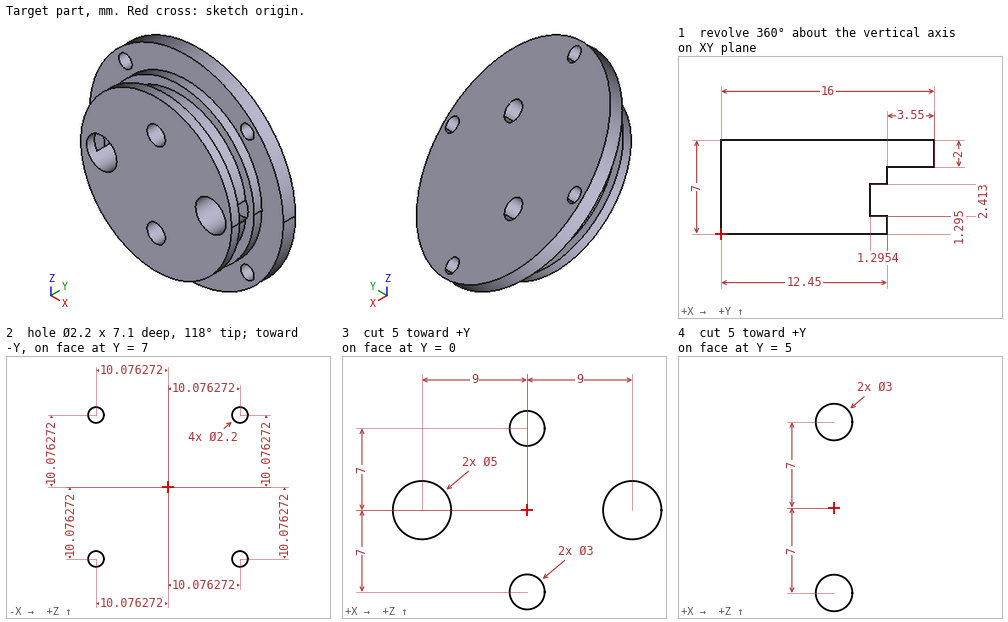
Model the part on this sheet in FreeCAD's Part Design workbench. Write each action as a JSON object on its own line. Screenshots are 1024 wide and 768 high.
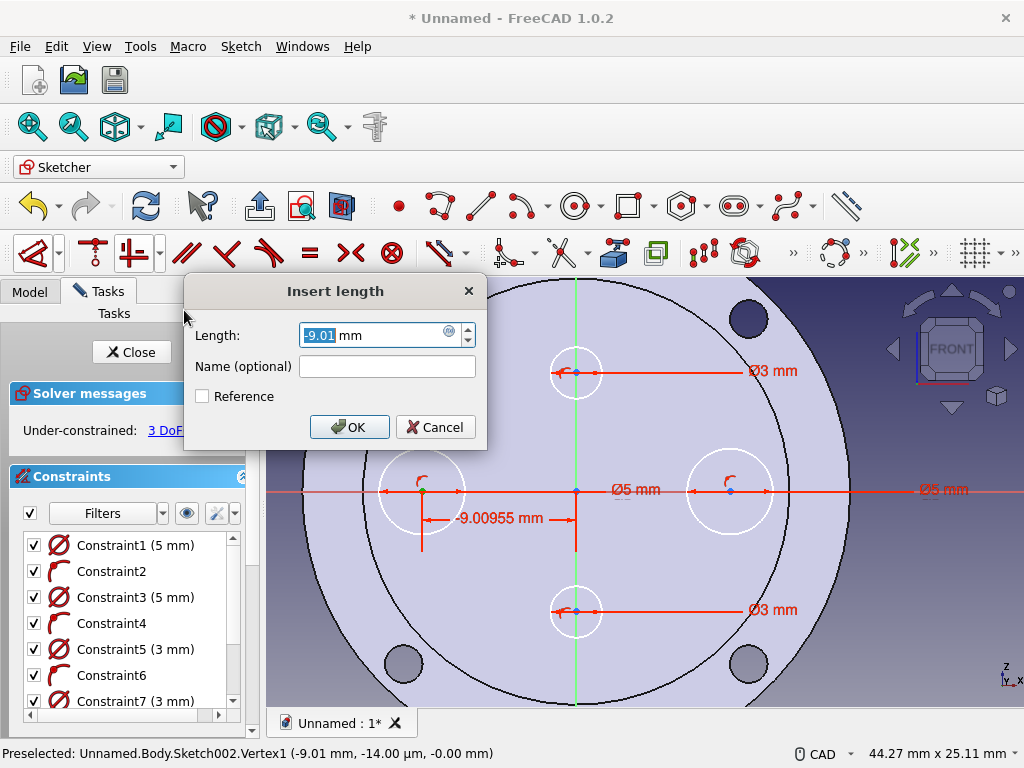
{"action": "type", "text": "-9"}
{"action": "key", "text": "Return"}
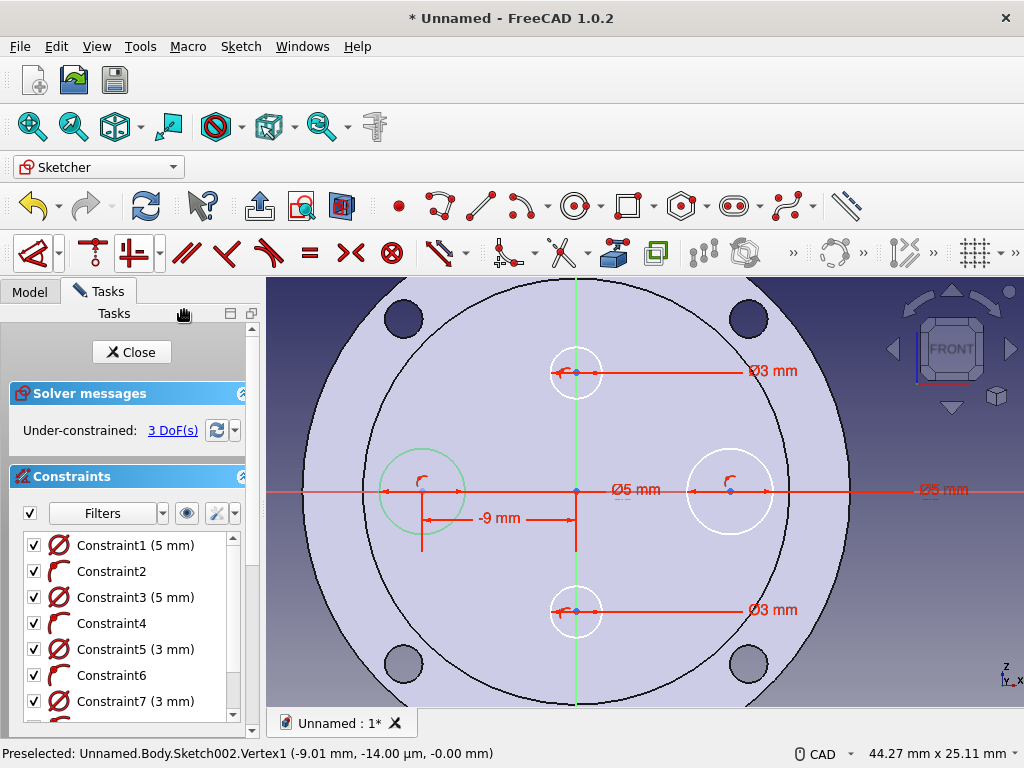
{"action": "left_click", "coordinate": [730, 492]}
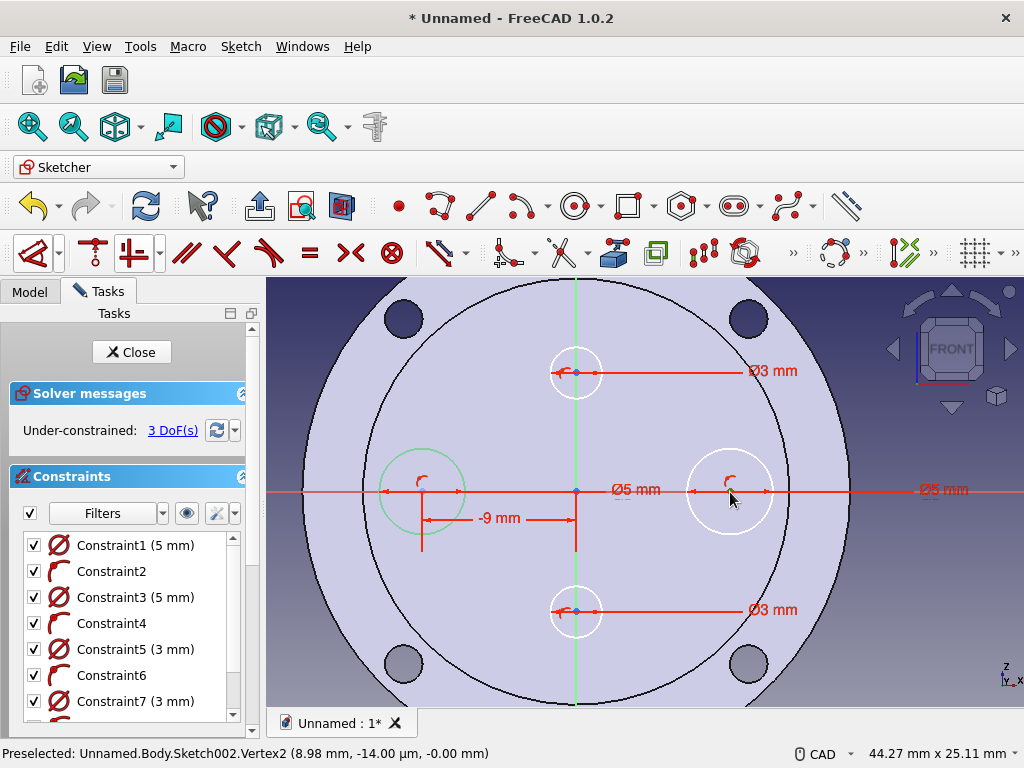
{"action": "key", "text": "l"}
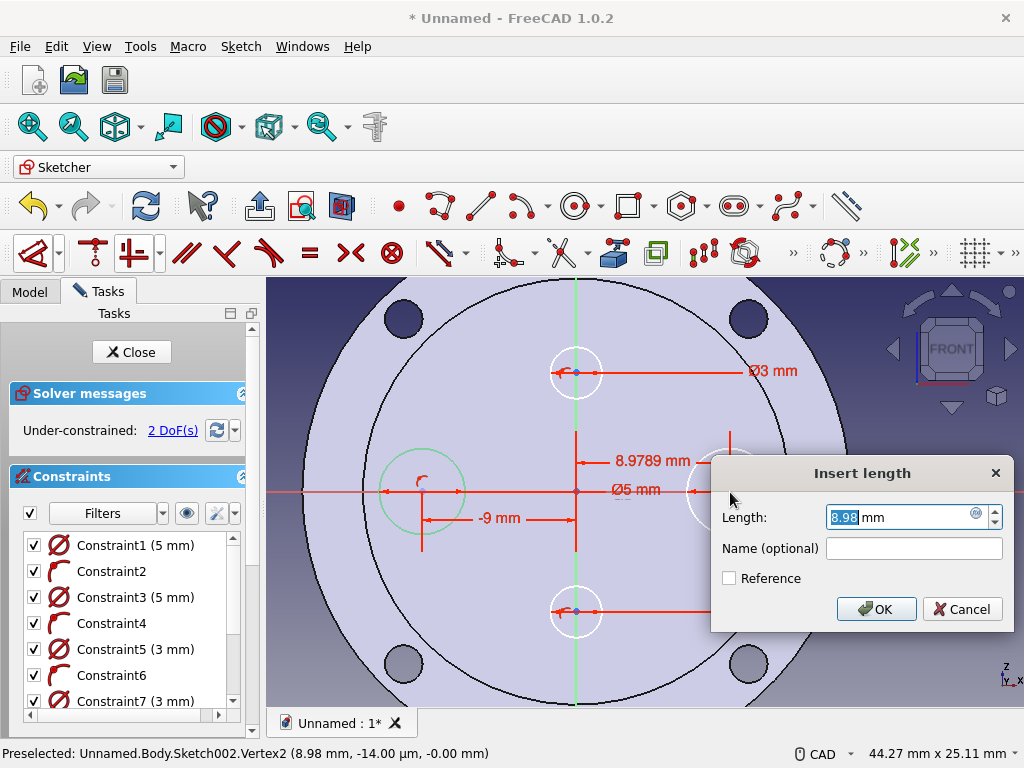
{"action": "type", "text": "9"}
{"action": "key", "text": "Return"}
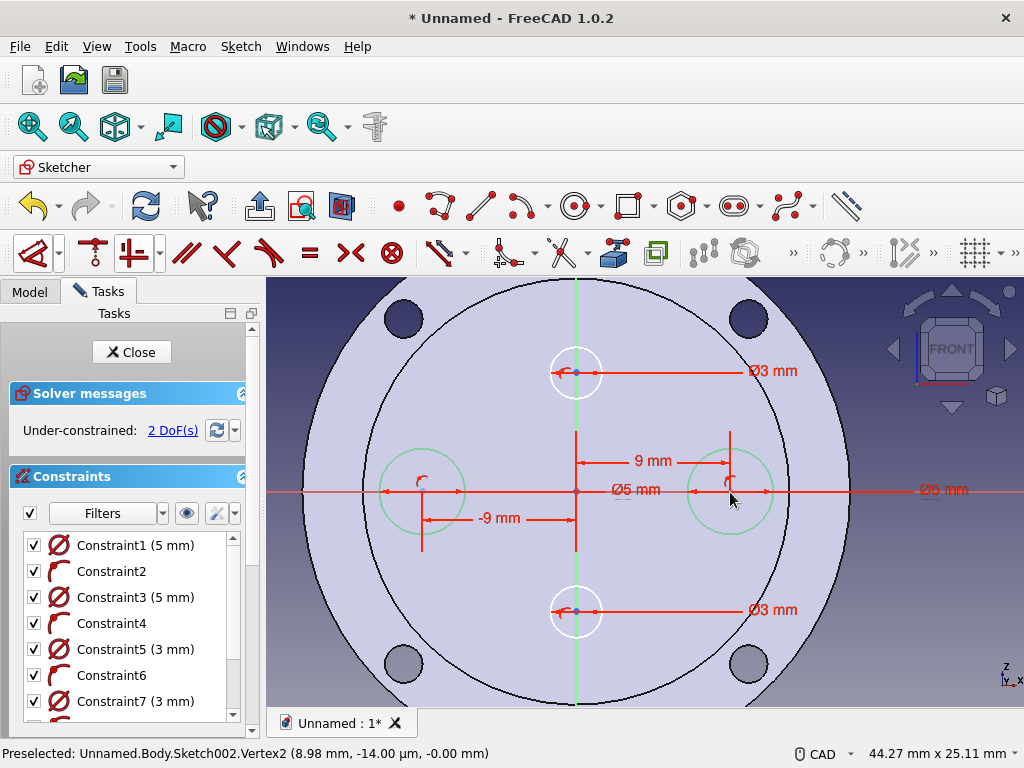
{"action": "left_click", "coordinate": [576, 612]}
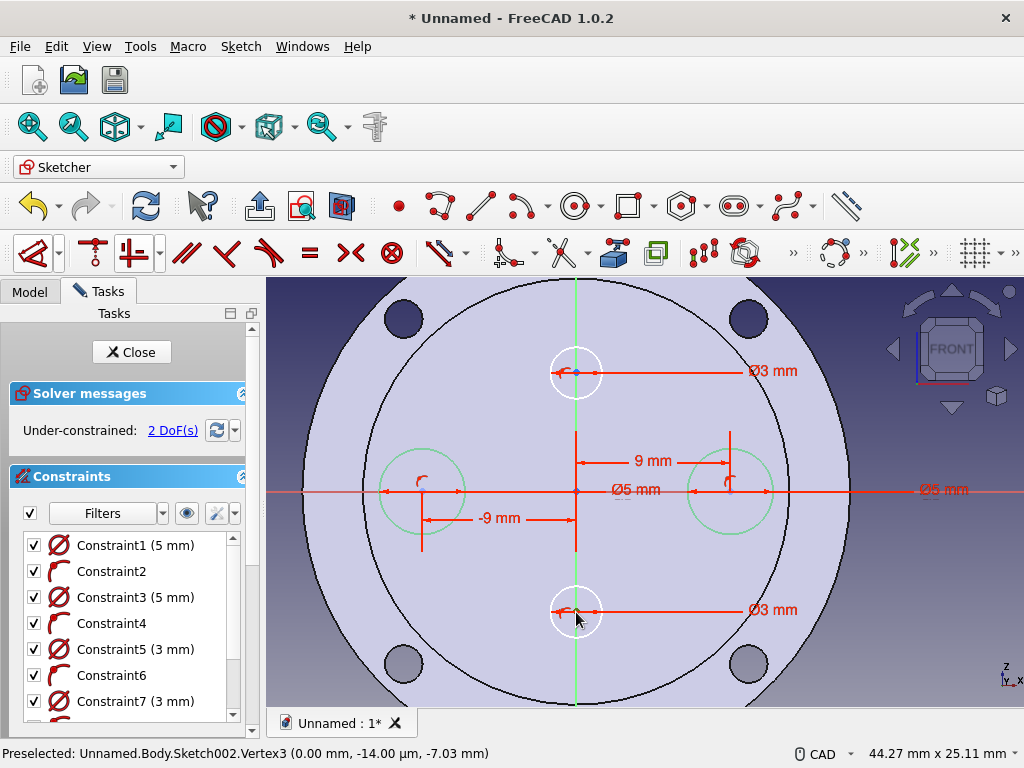
{"action": "left_click", "coordinate": [58, 254]}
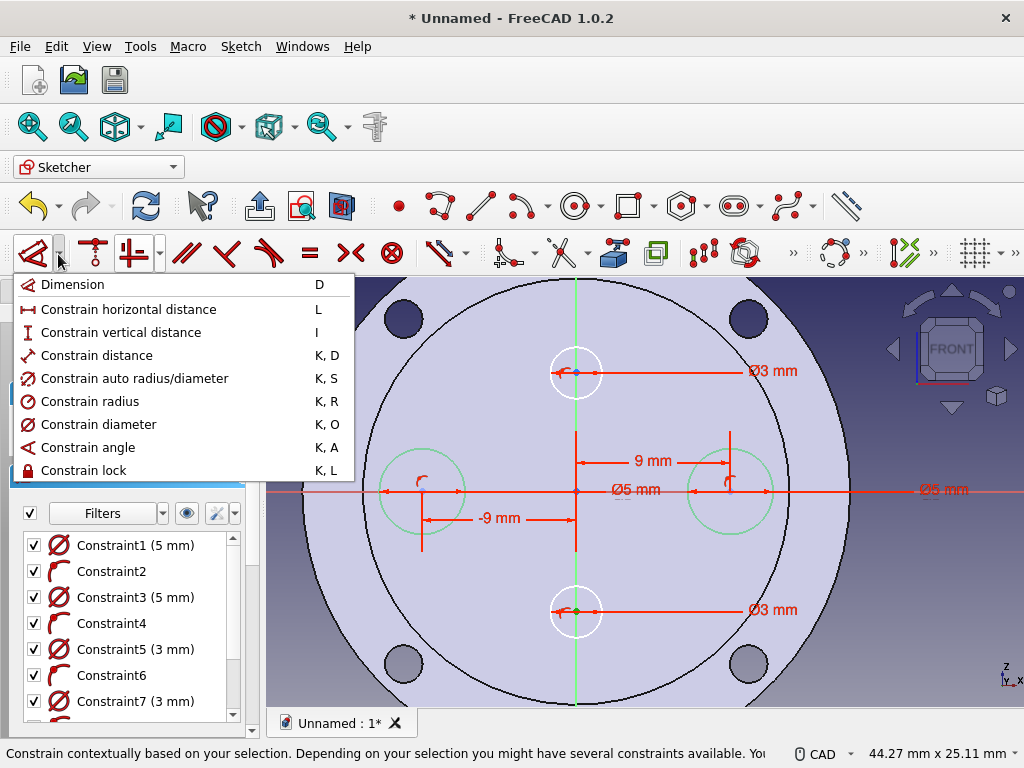
{"action": "left_click", "coordinate": [184, 332]}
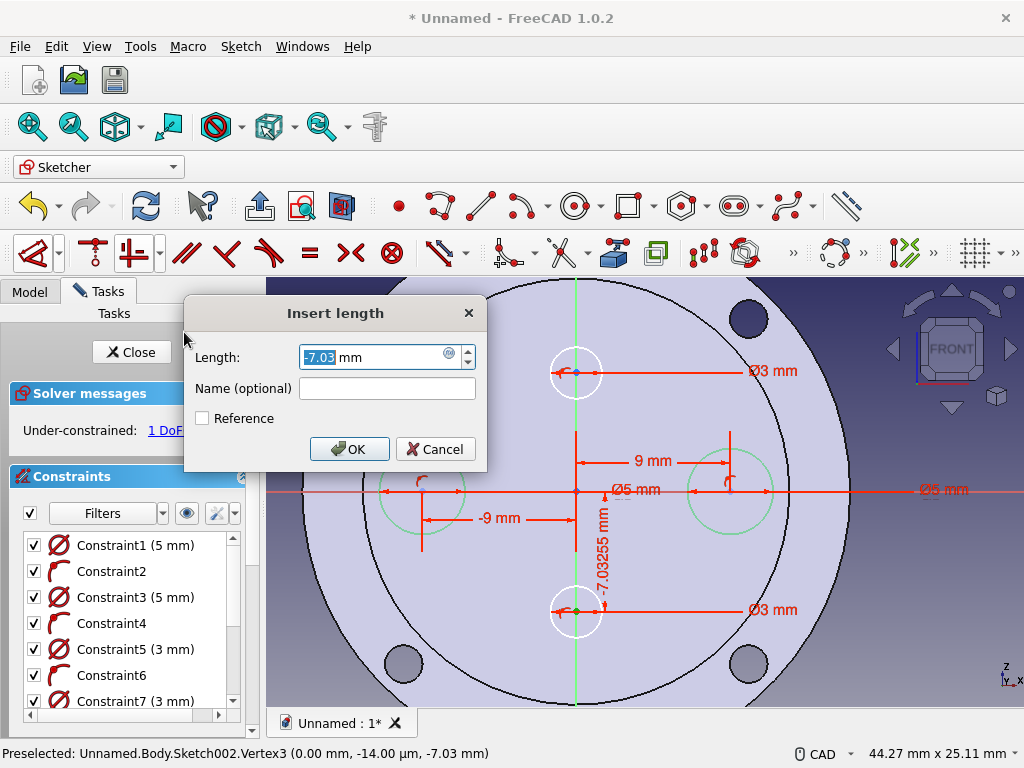
{"action": "type", "text": "-7"}
{"action": "key", "text": "Return"}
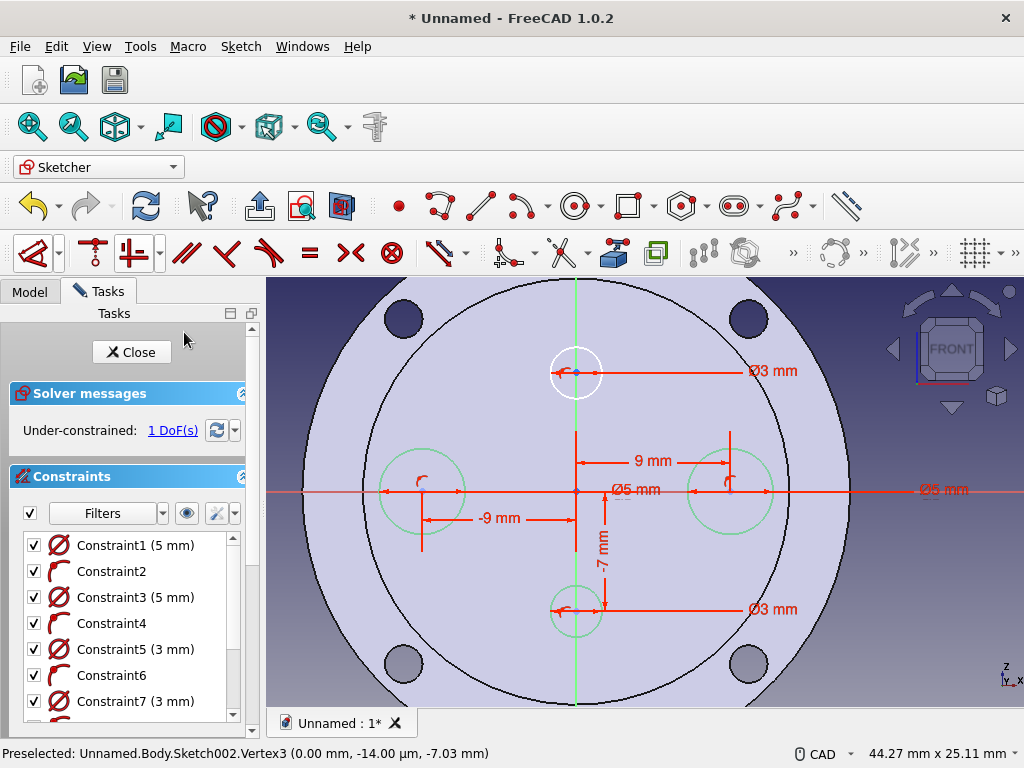
{"action": "left_click", "coordinate": [576, 373]}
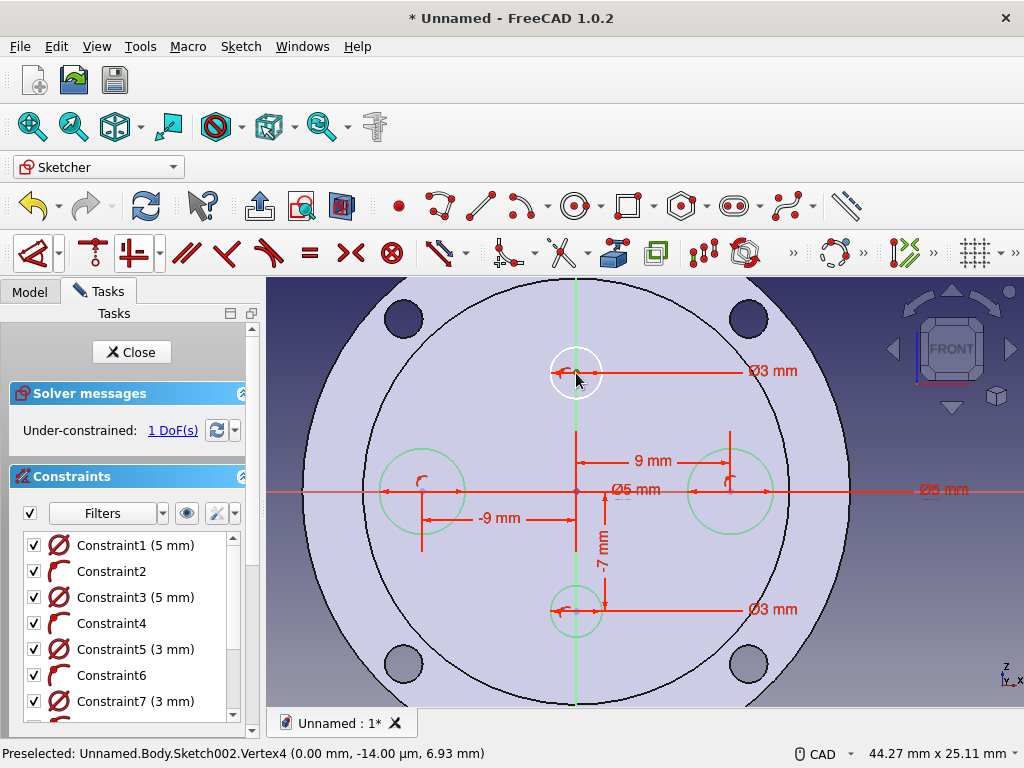
{"action": "left_click", "coordinate": [58, 254]}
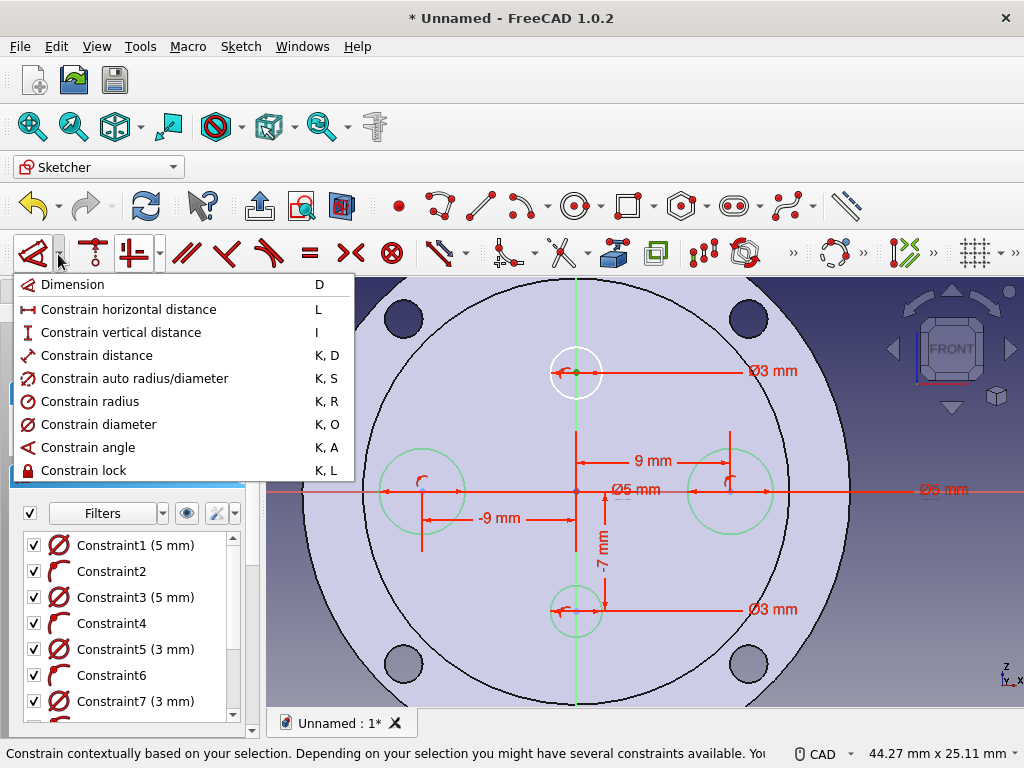
{"action": "left_click", "coordinate": [184, 332]}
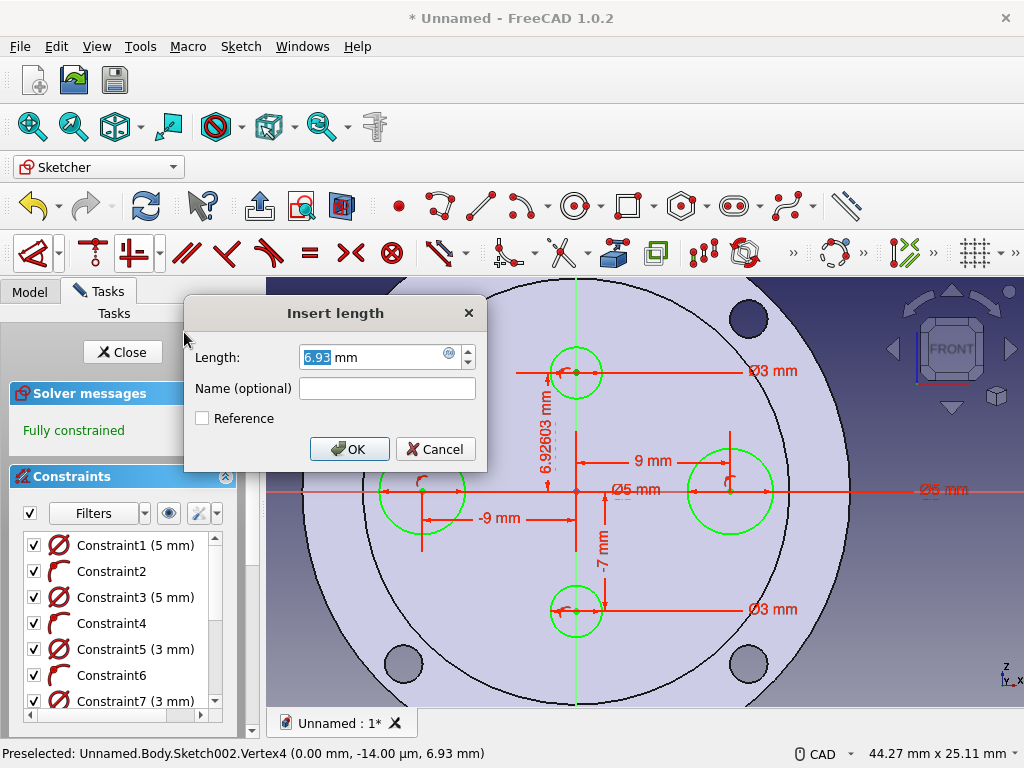
{"action": "type", "text": "7"}
{"action": "key", "text": "Return"}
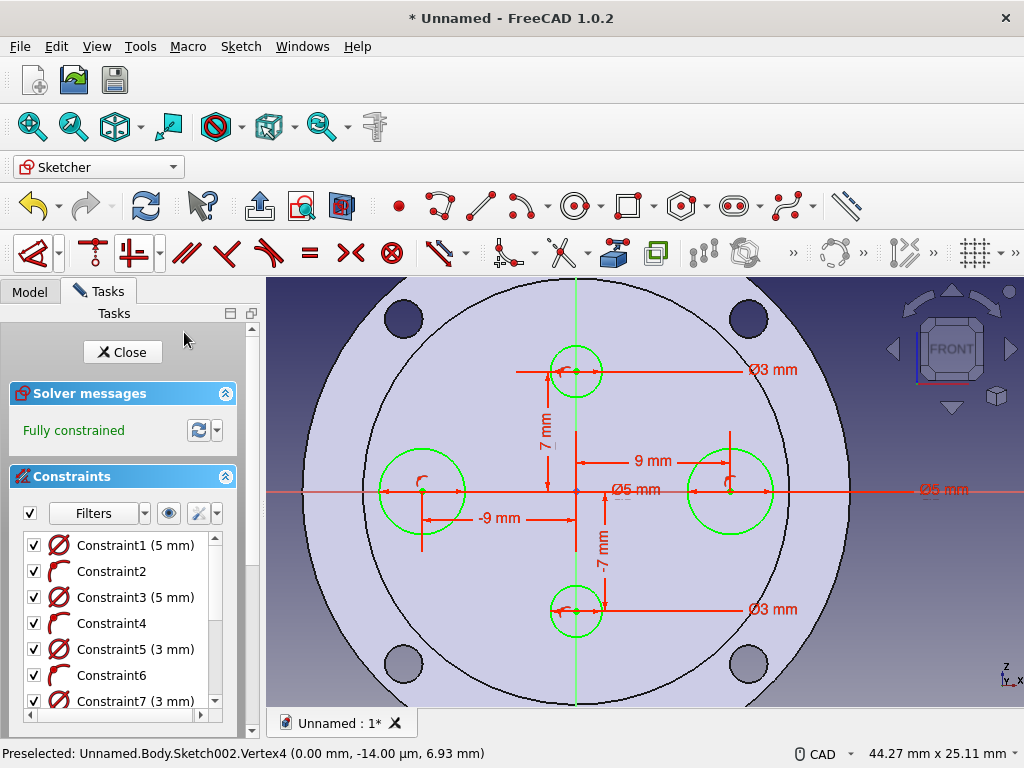
{"action": "left_click", "coordinate": [123, 352]}